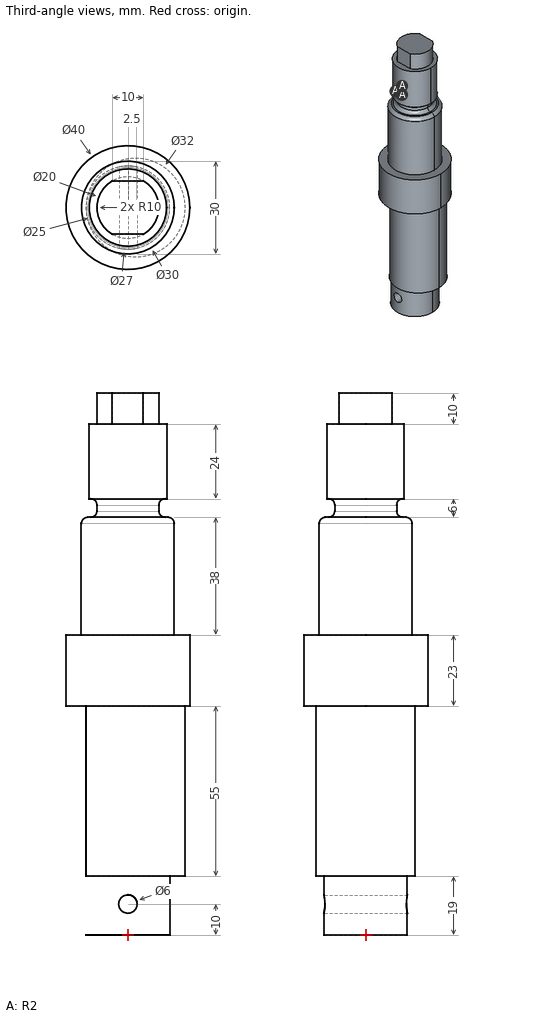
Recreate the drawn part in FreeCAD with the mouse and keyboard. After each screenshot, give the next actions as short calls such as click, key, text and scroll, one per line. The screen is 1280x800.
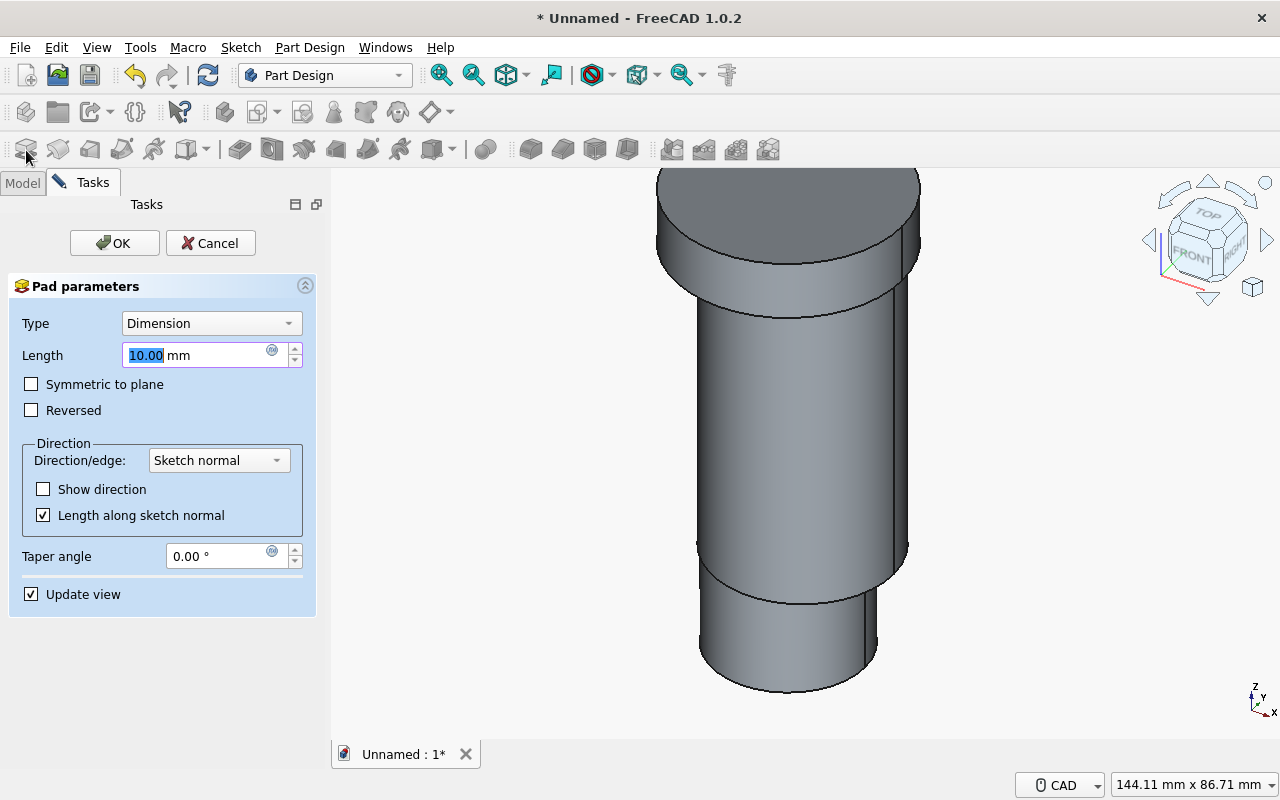
text(23)
key(Tab)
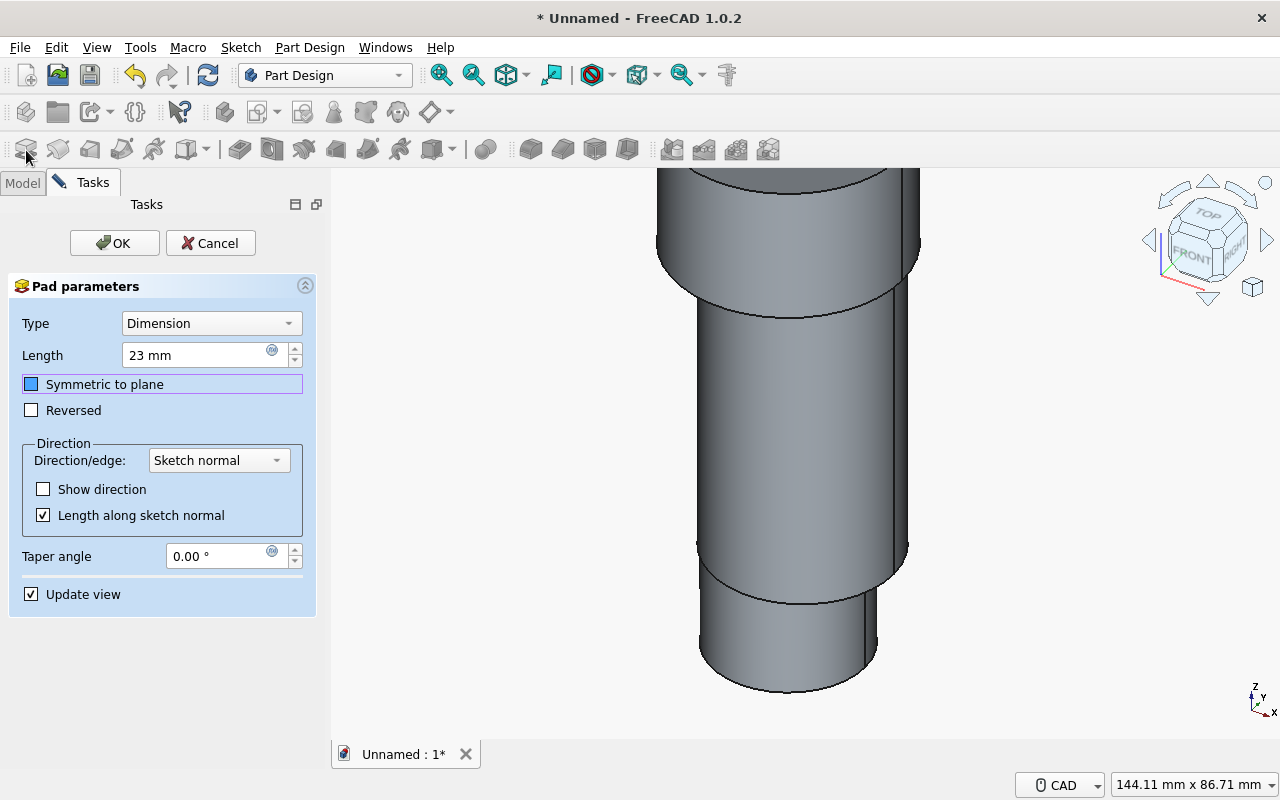
click(115, 243)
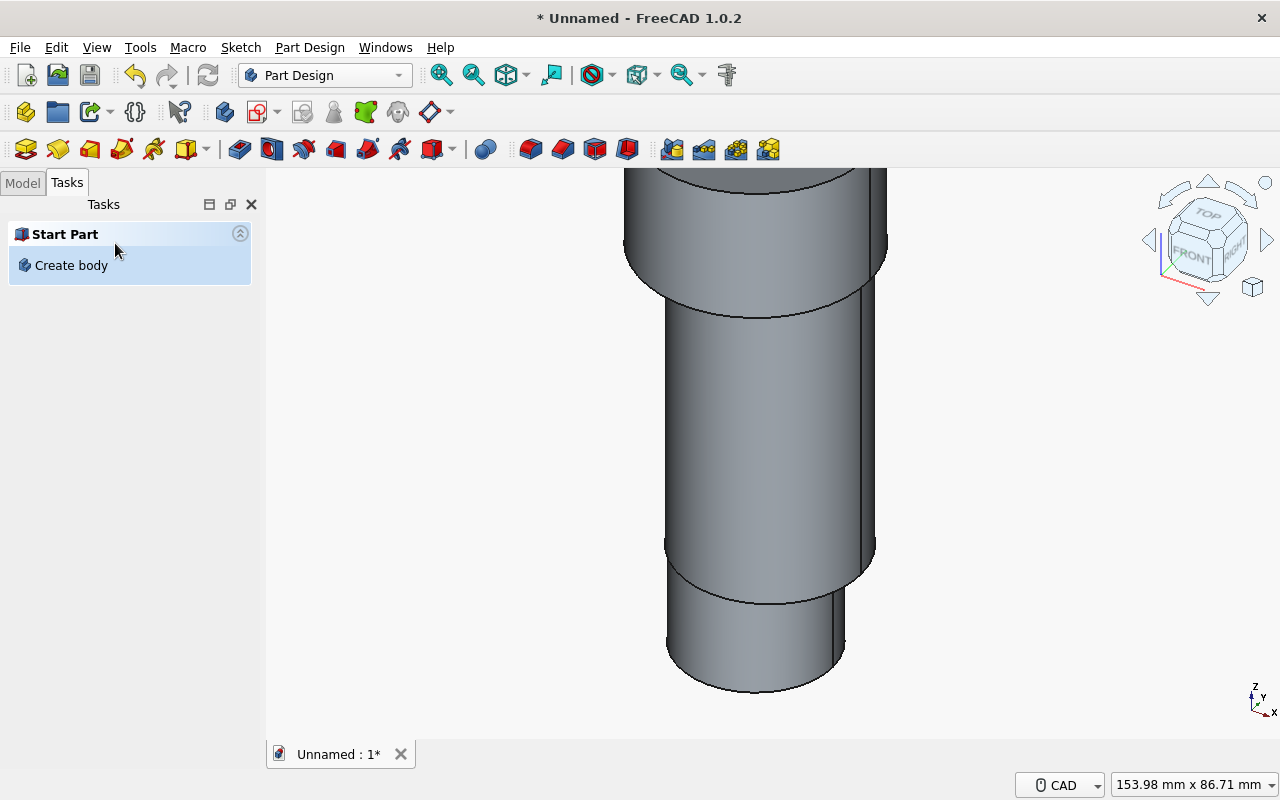
key(v)
key(f)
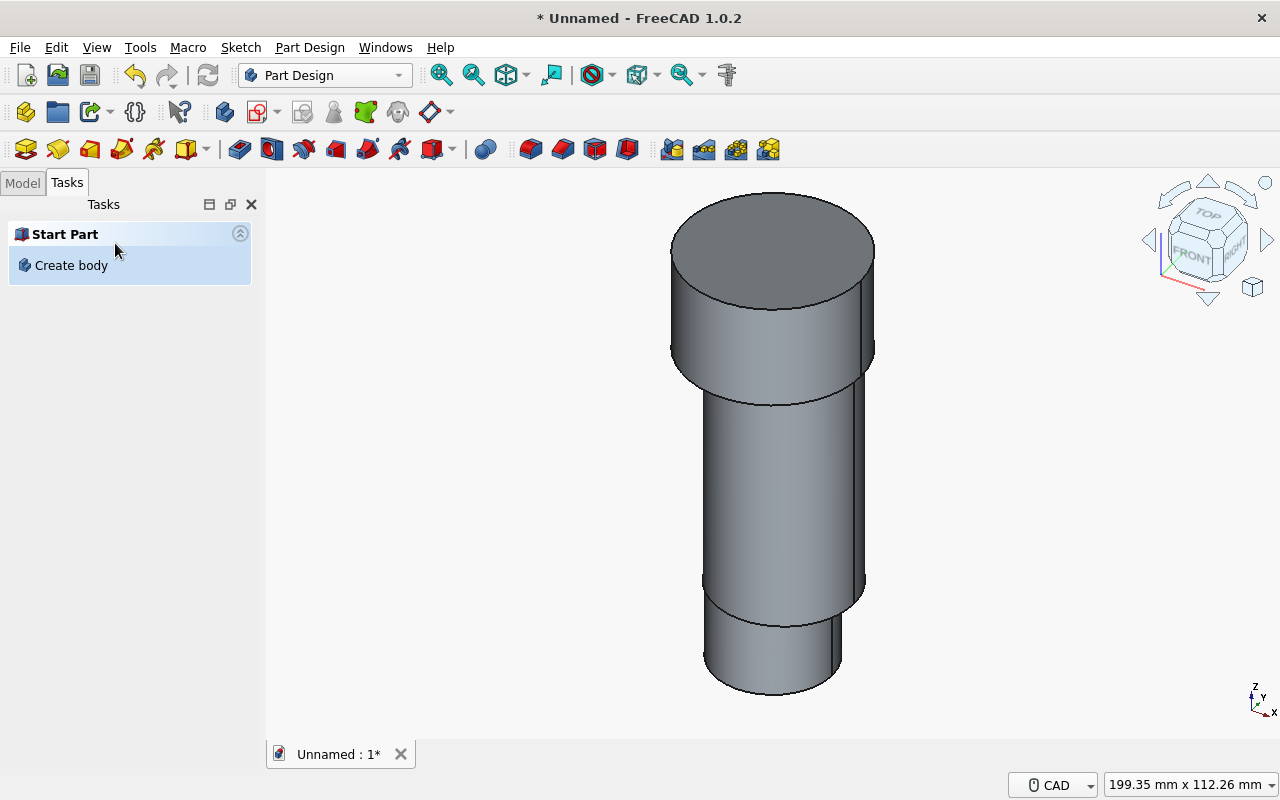
click(773, 250)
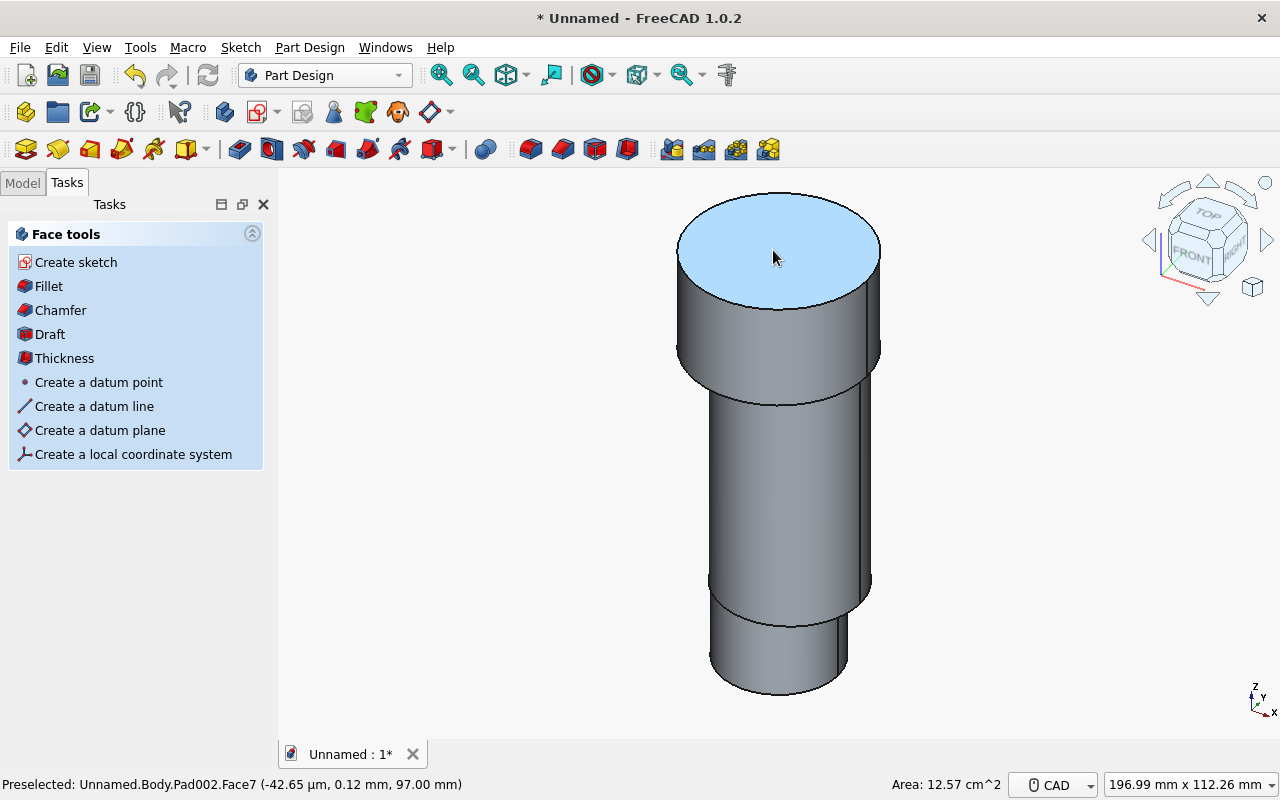
click(258, 112)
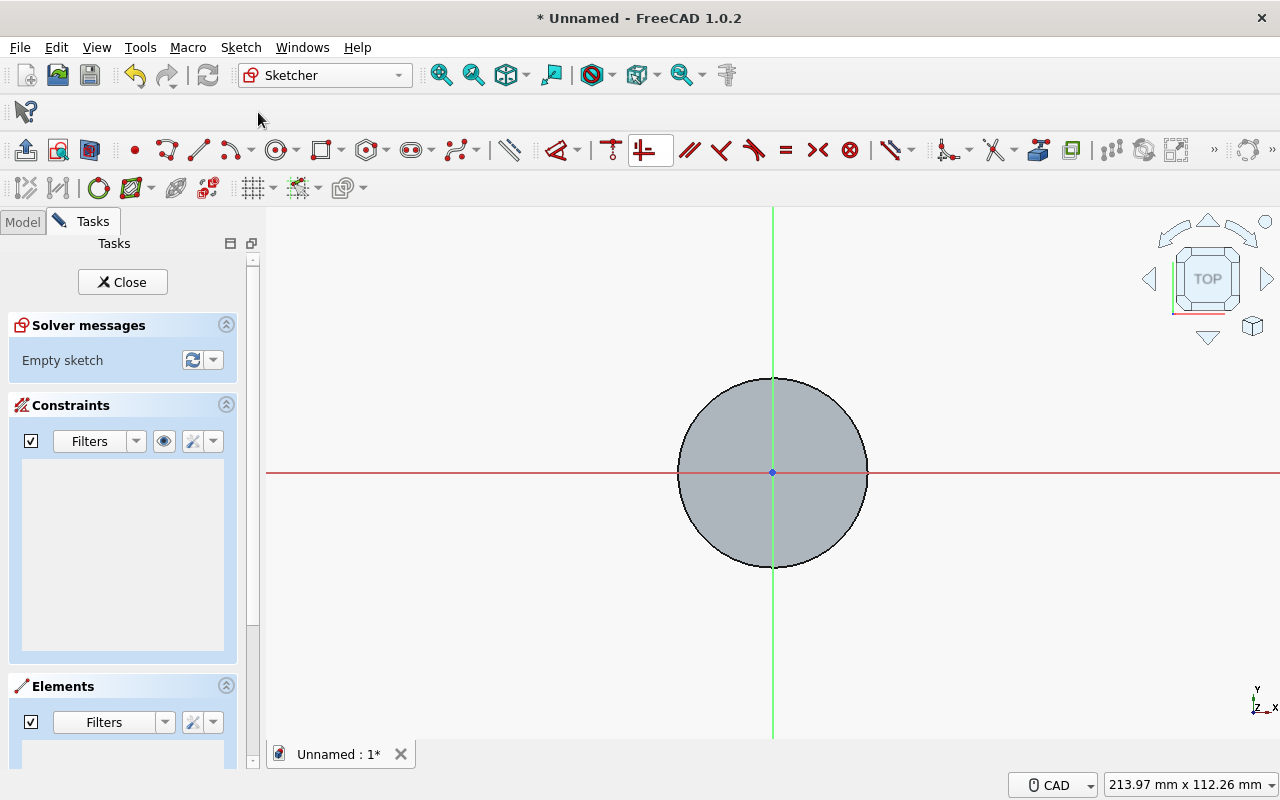
scroll(829, 473, up, 4)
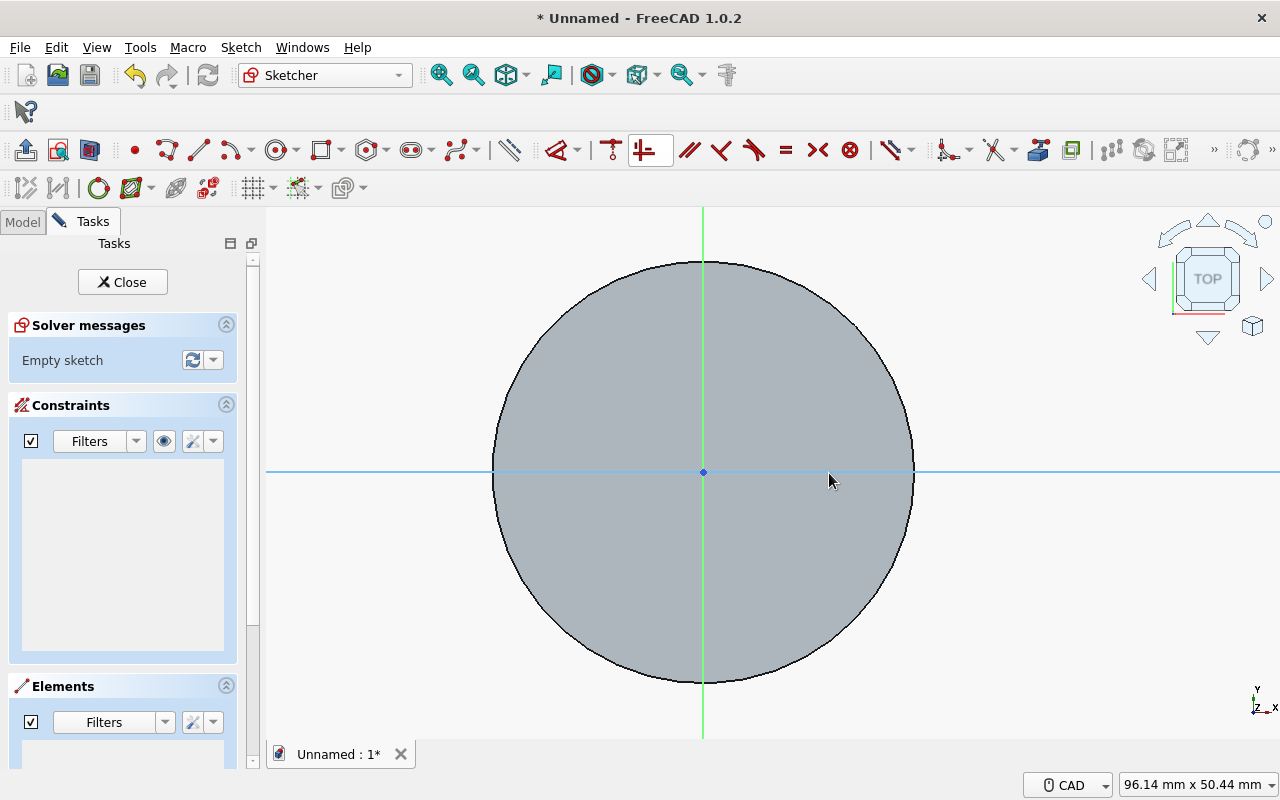
key(g)
key(c)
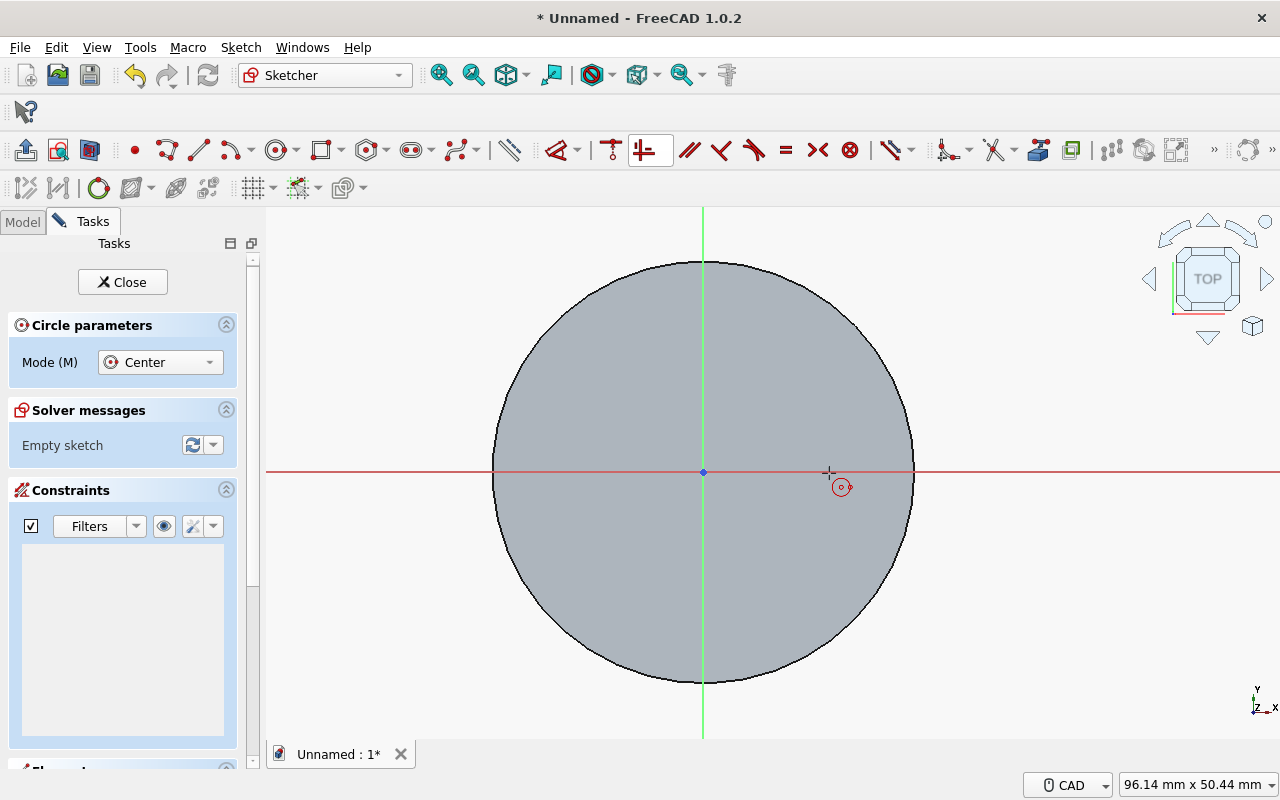
click(703, 472)
click(815, 361)
key(Escape)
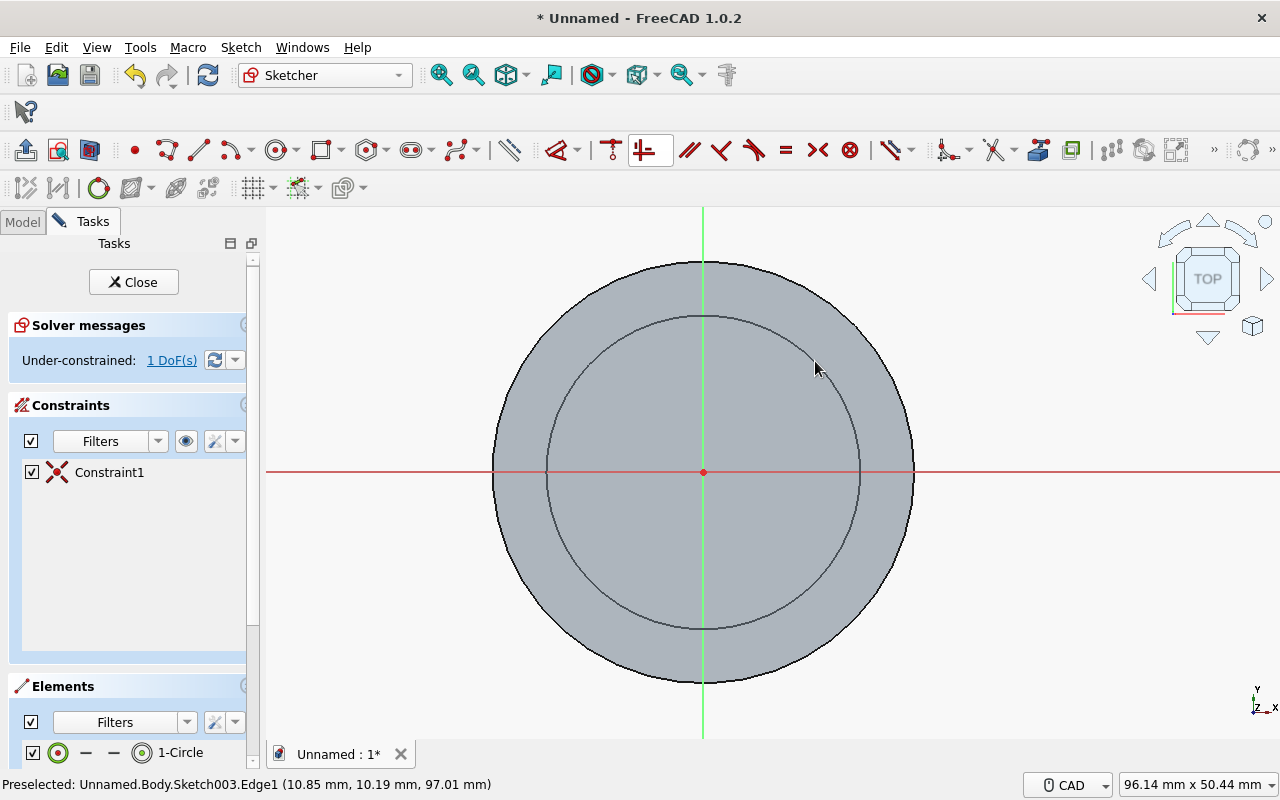
key(d)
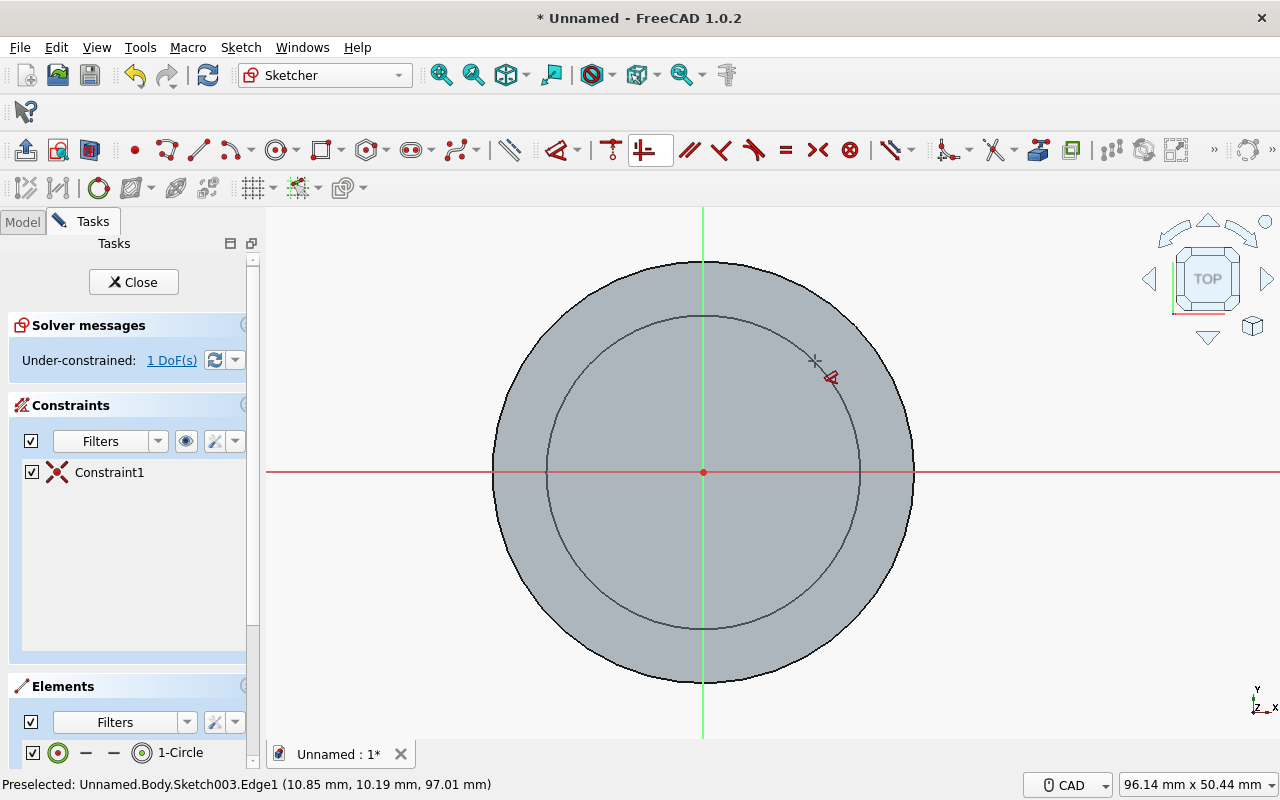
click(814, 361)
click(837, 338)